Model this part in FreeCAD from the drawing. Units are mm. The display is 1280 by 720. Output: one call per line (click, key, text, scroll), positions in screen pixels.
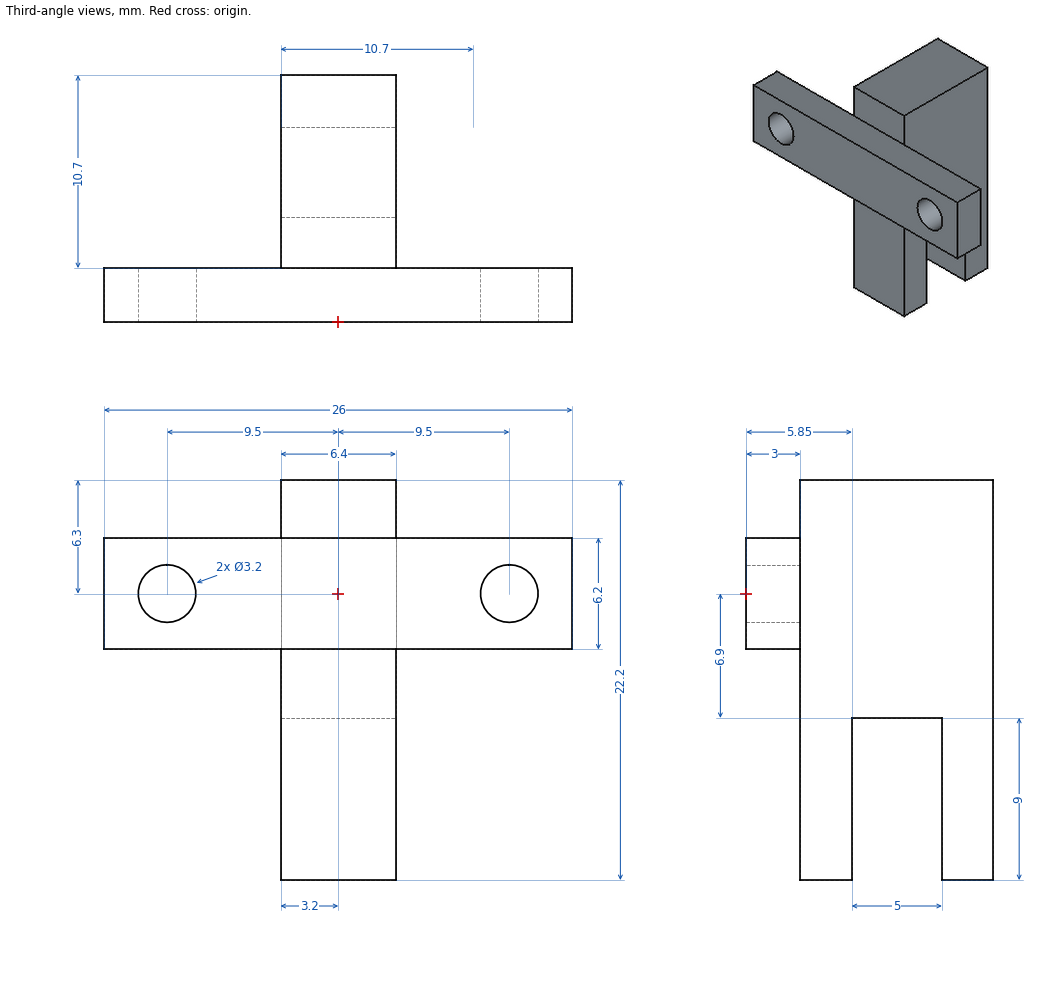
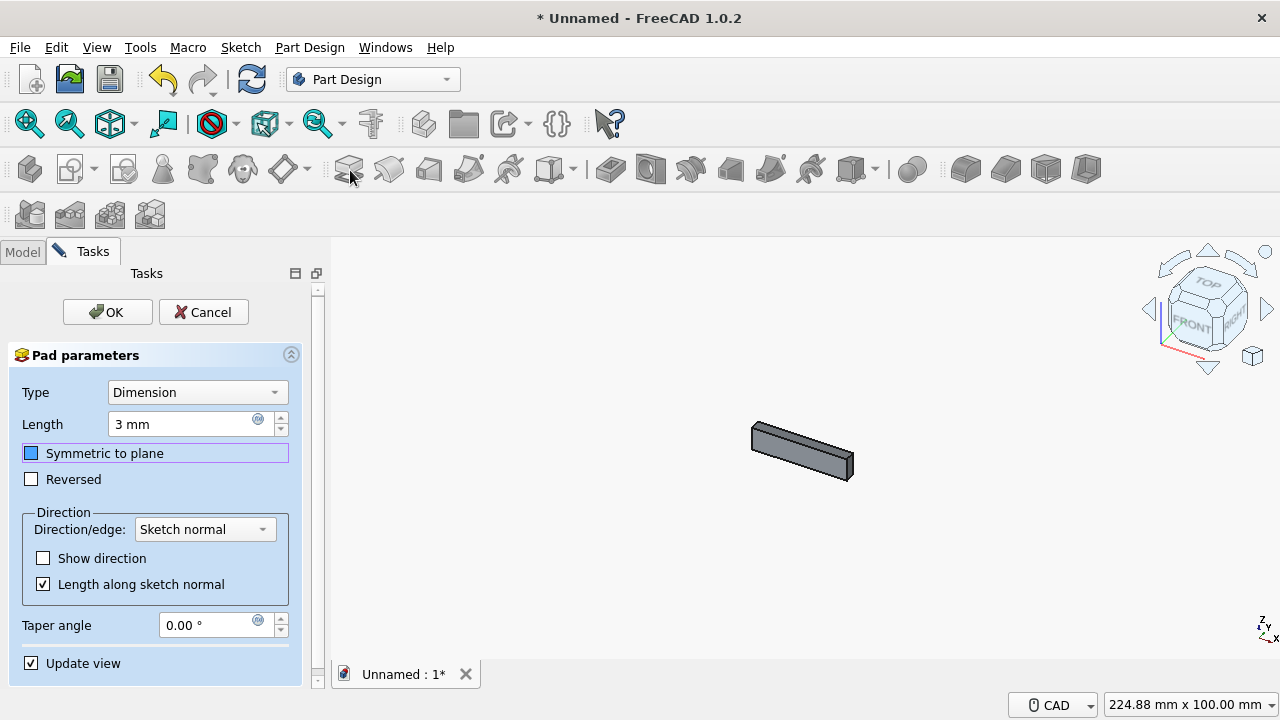
click(30, 479)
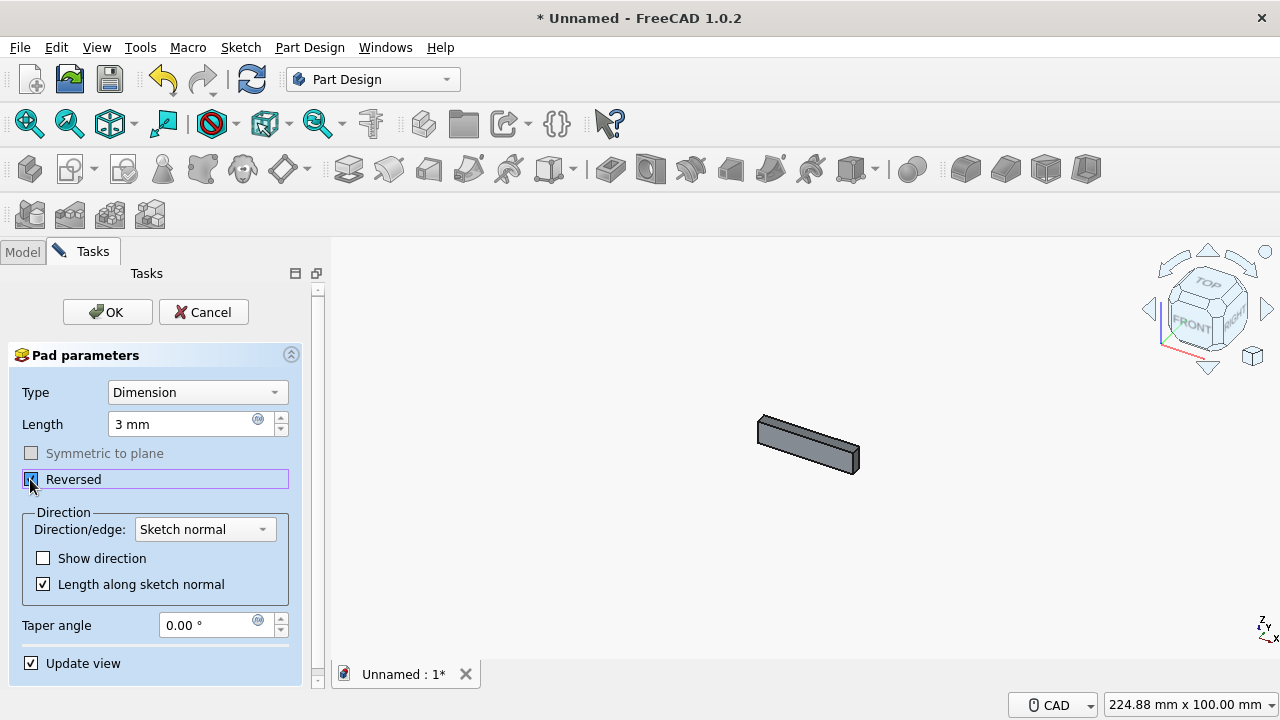
click(108, 312)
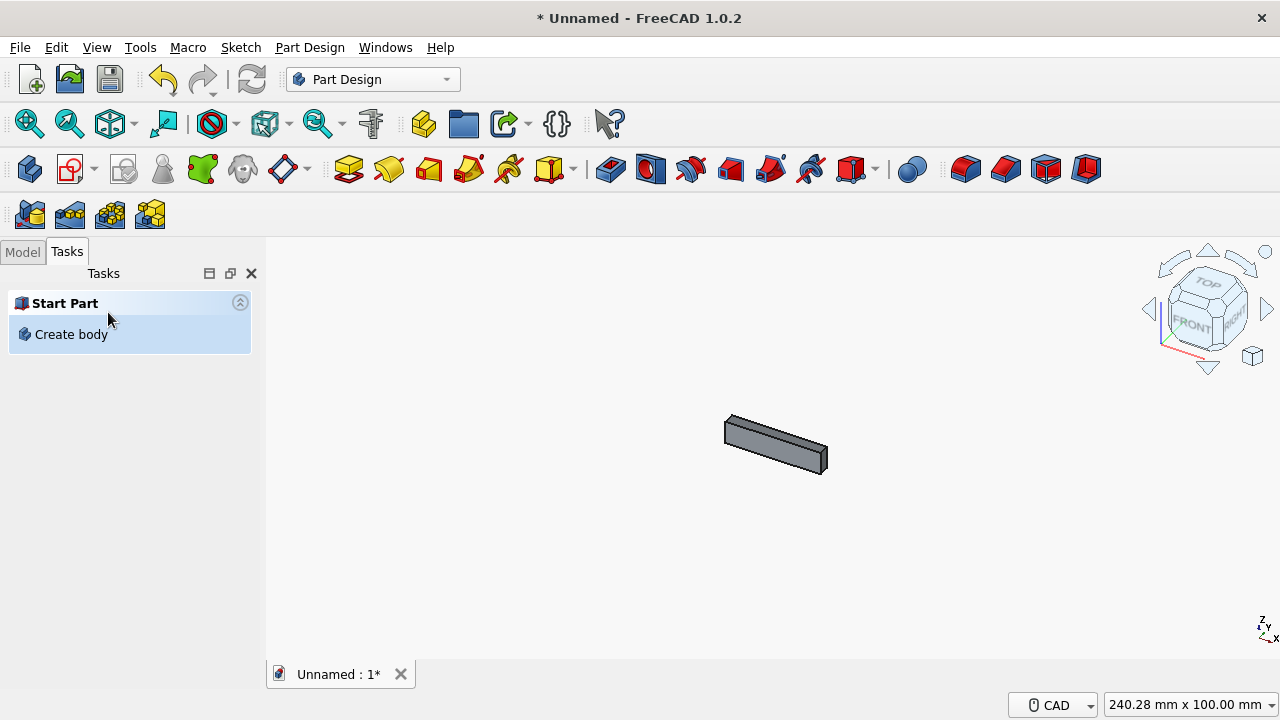
key(v)
key(f)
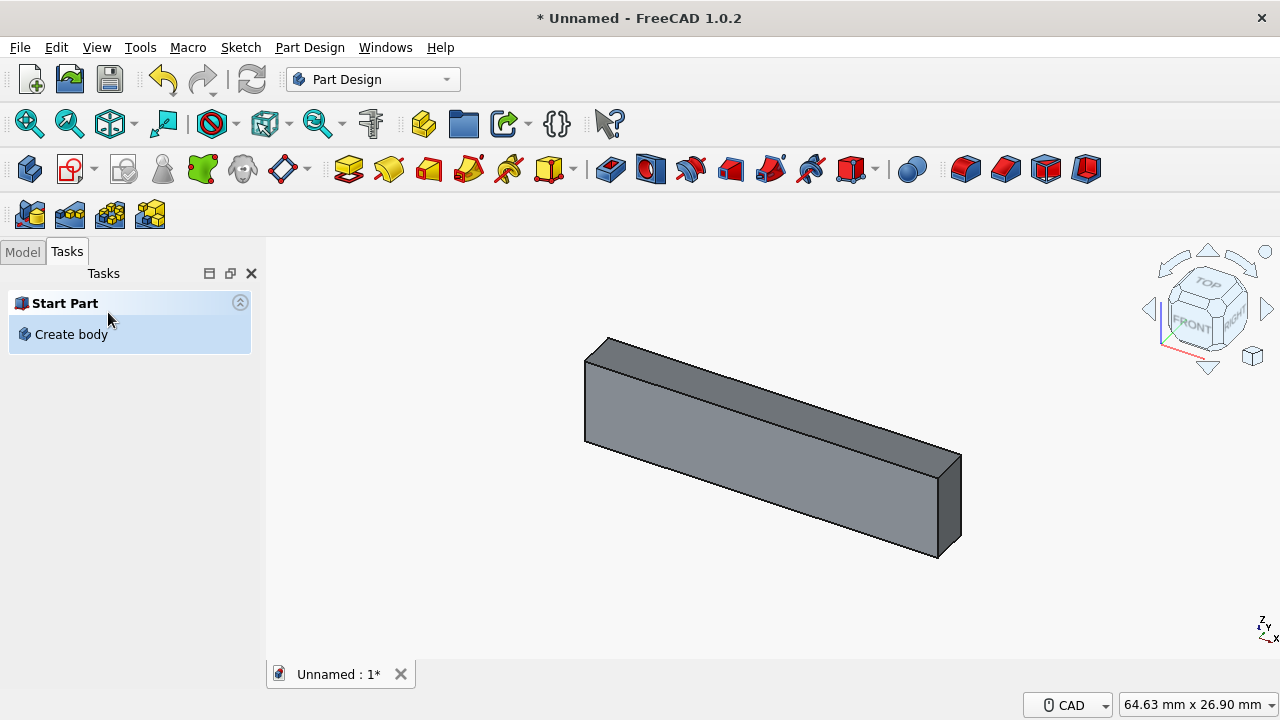
key(4)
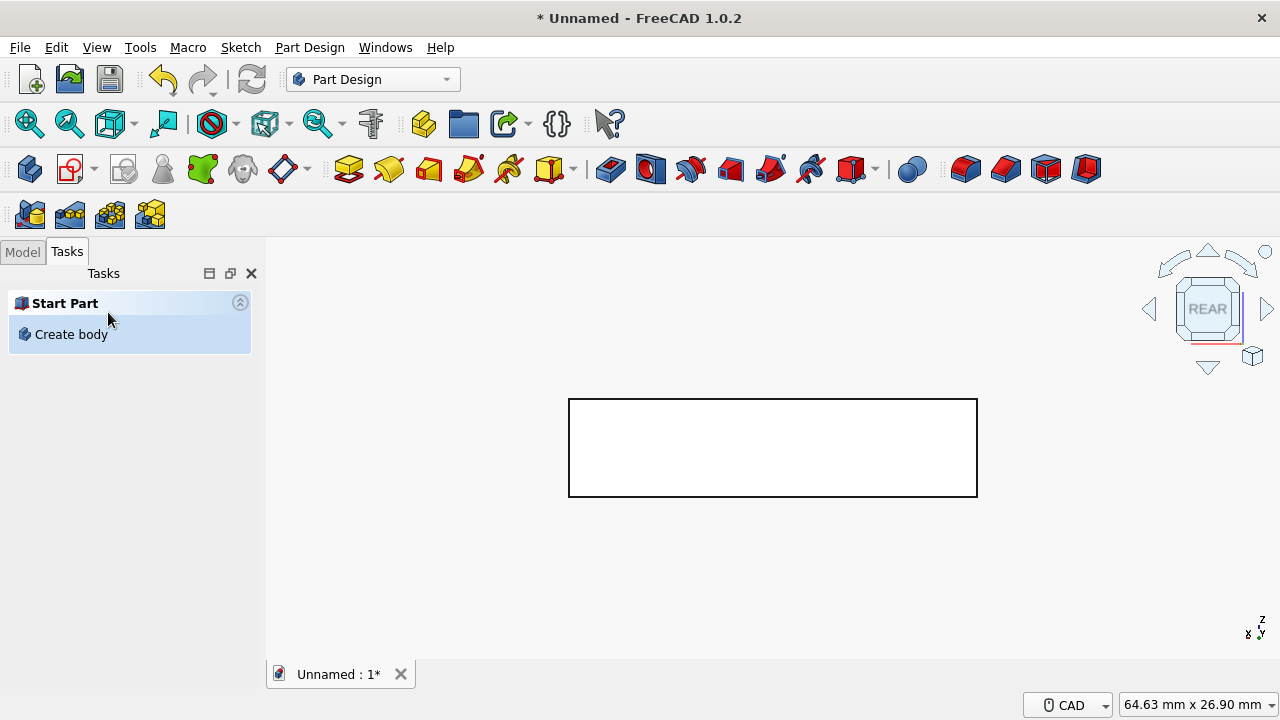
key(v)
key(f)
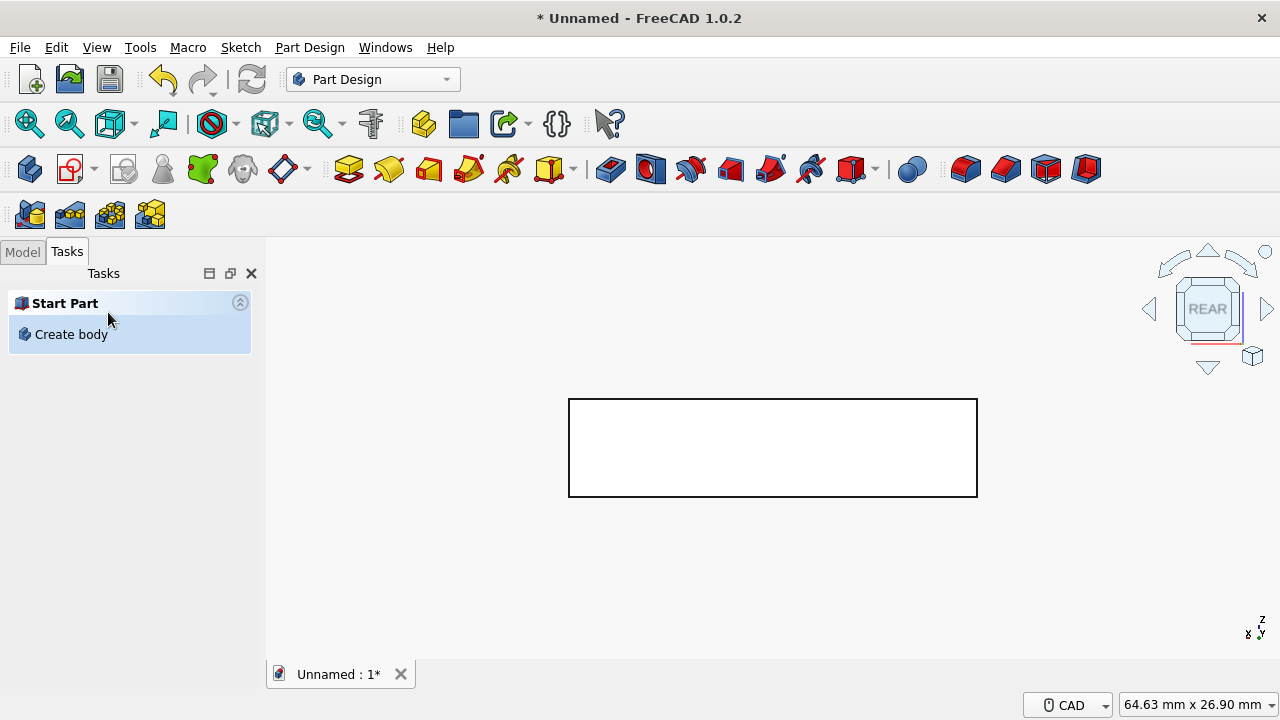
click(656, 447)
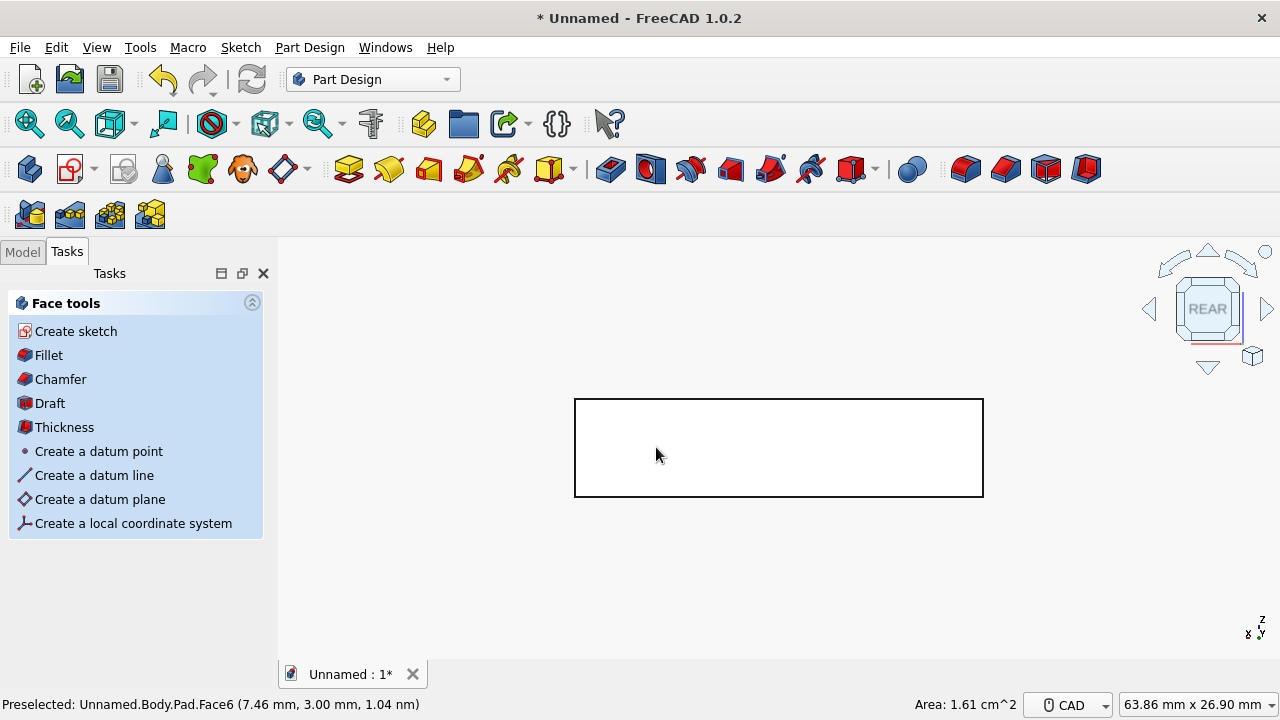
click(70, 170)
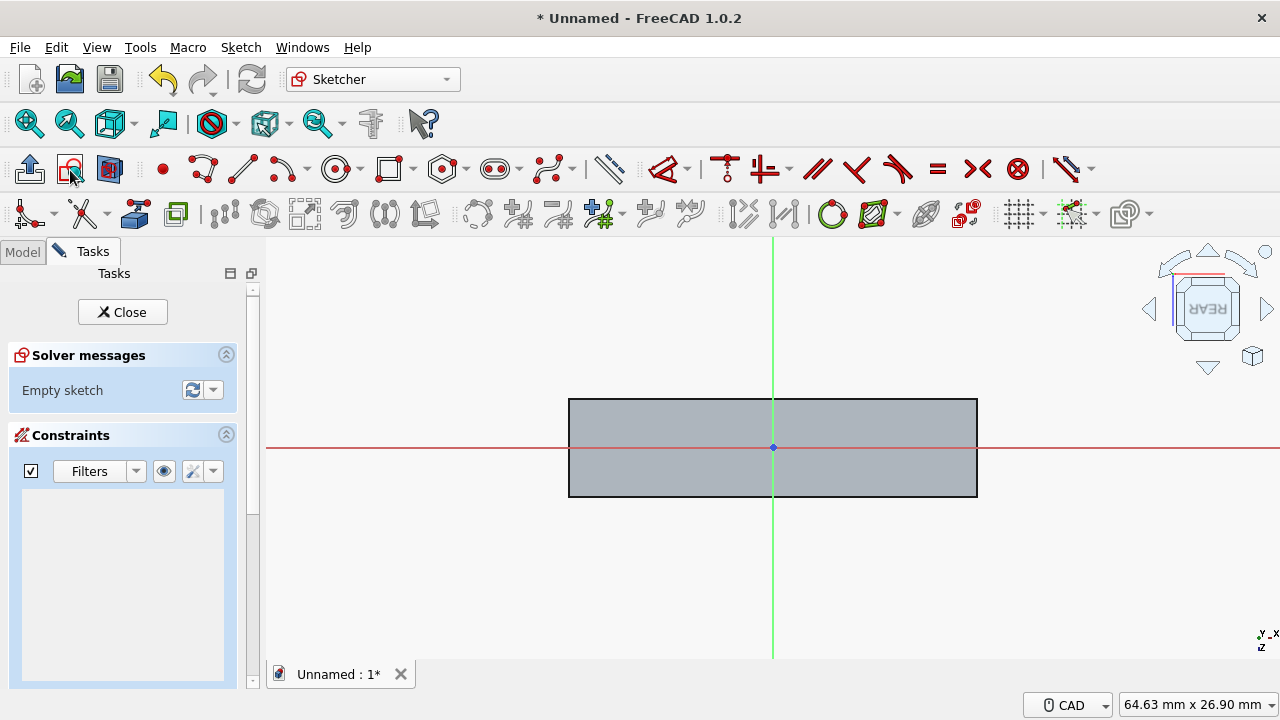
scroll(565, 601, down, 2)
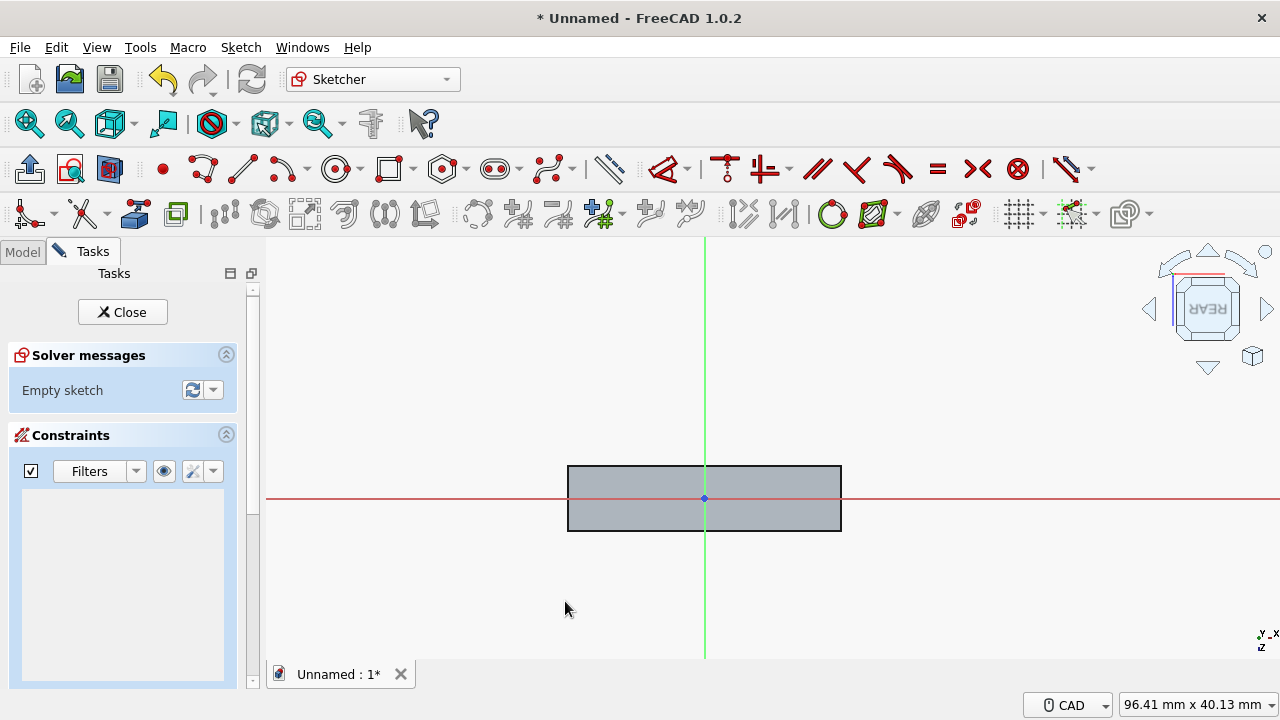
key(g)
key(r)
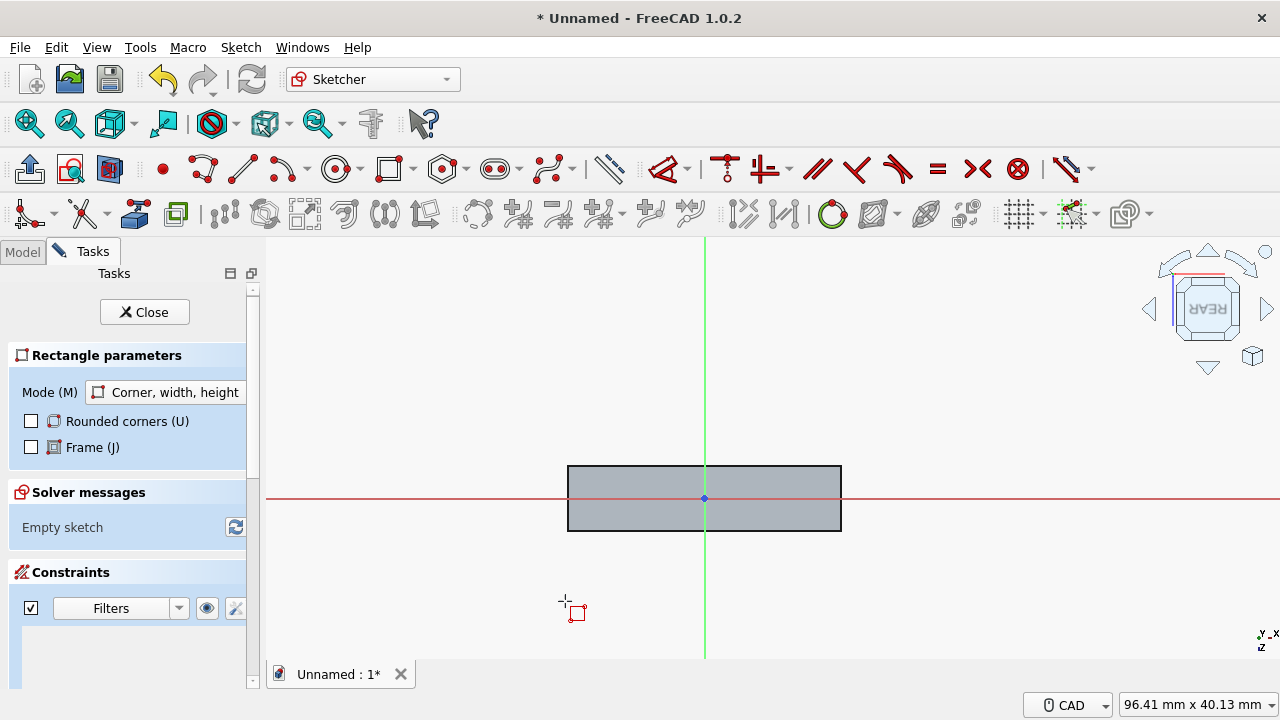
click(671, 332)
move(738, 565)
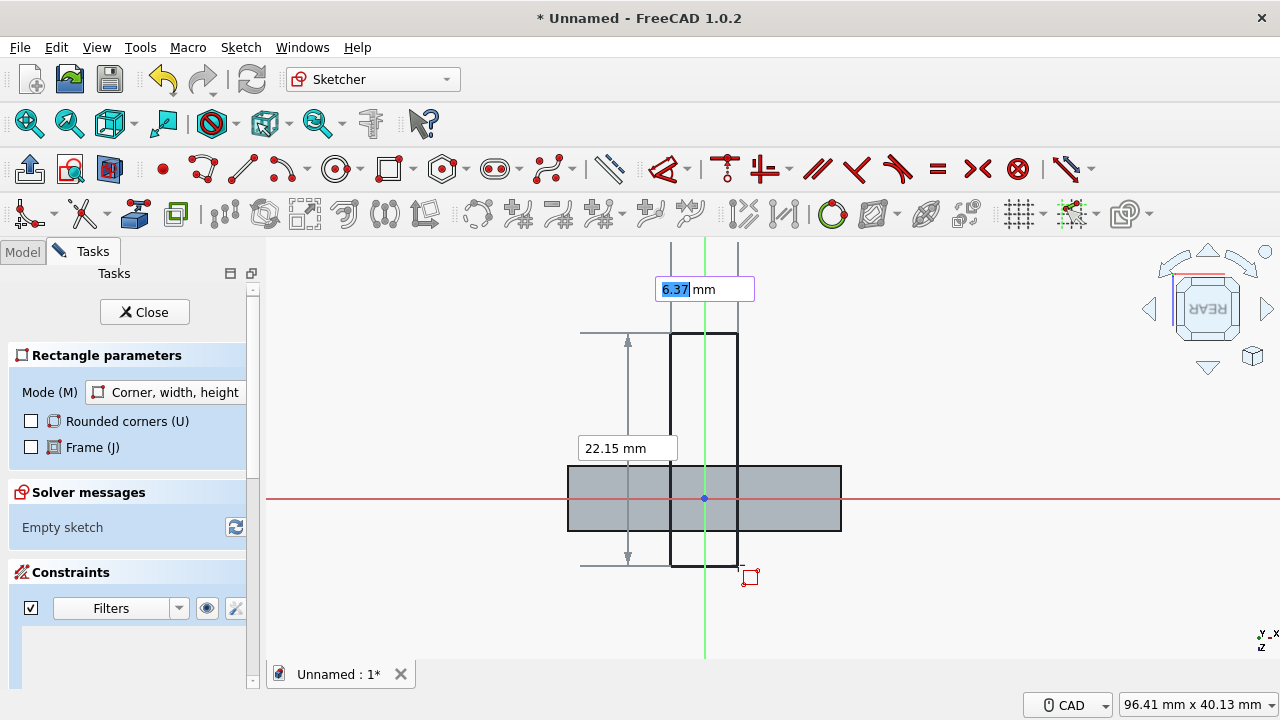
text(6.4)
key(Tab)
text(22.2)
key(Return)
key(Escape)